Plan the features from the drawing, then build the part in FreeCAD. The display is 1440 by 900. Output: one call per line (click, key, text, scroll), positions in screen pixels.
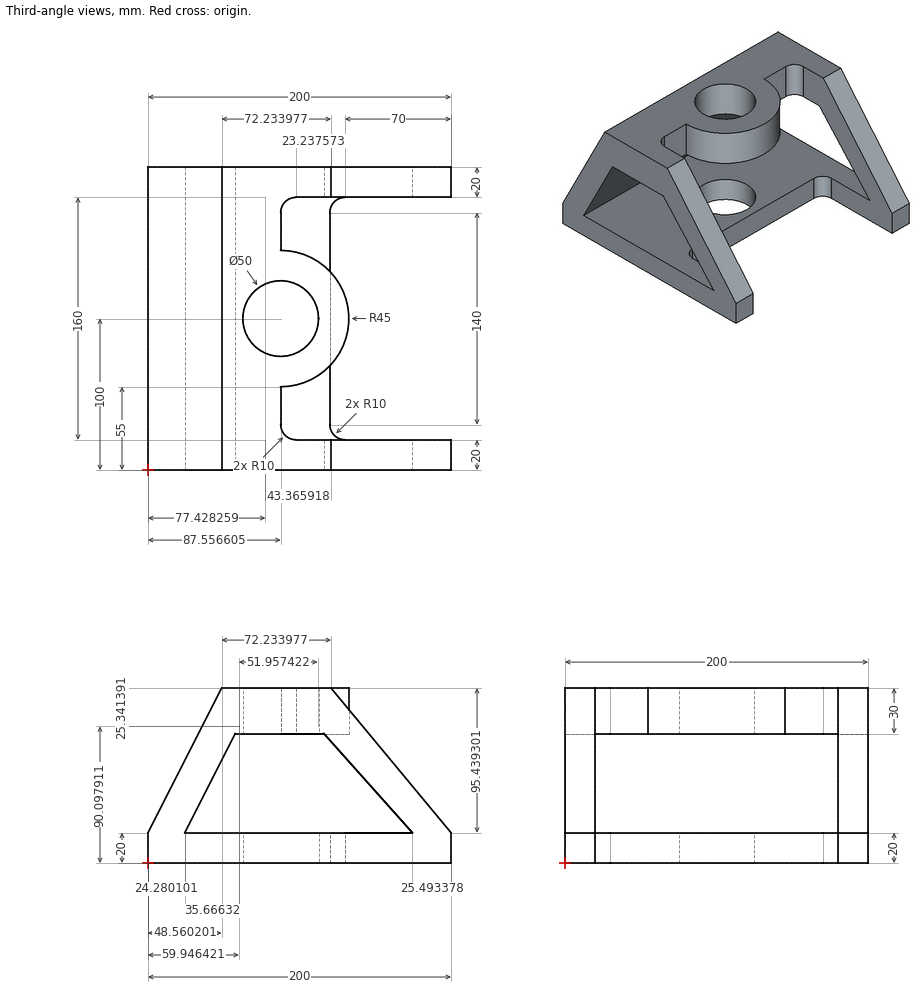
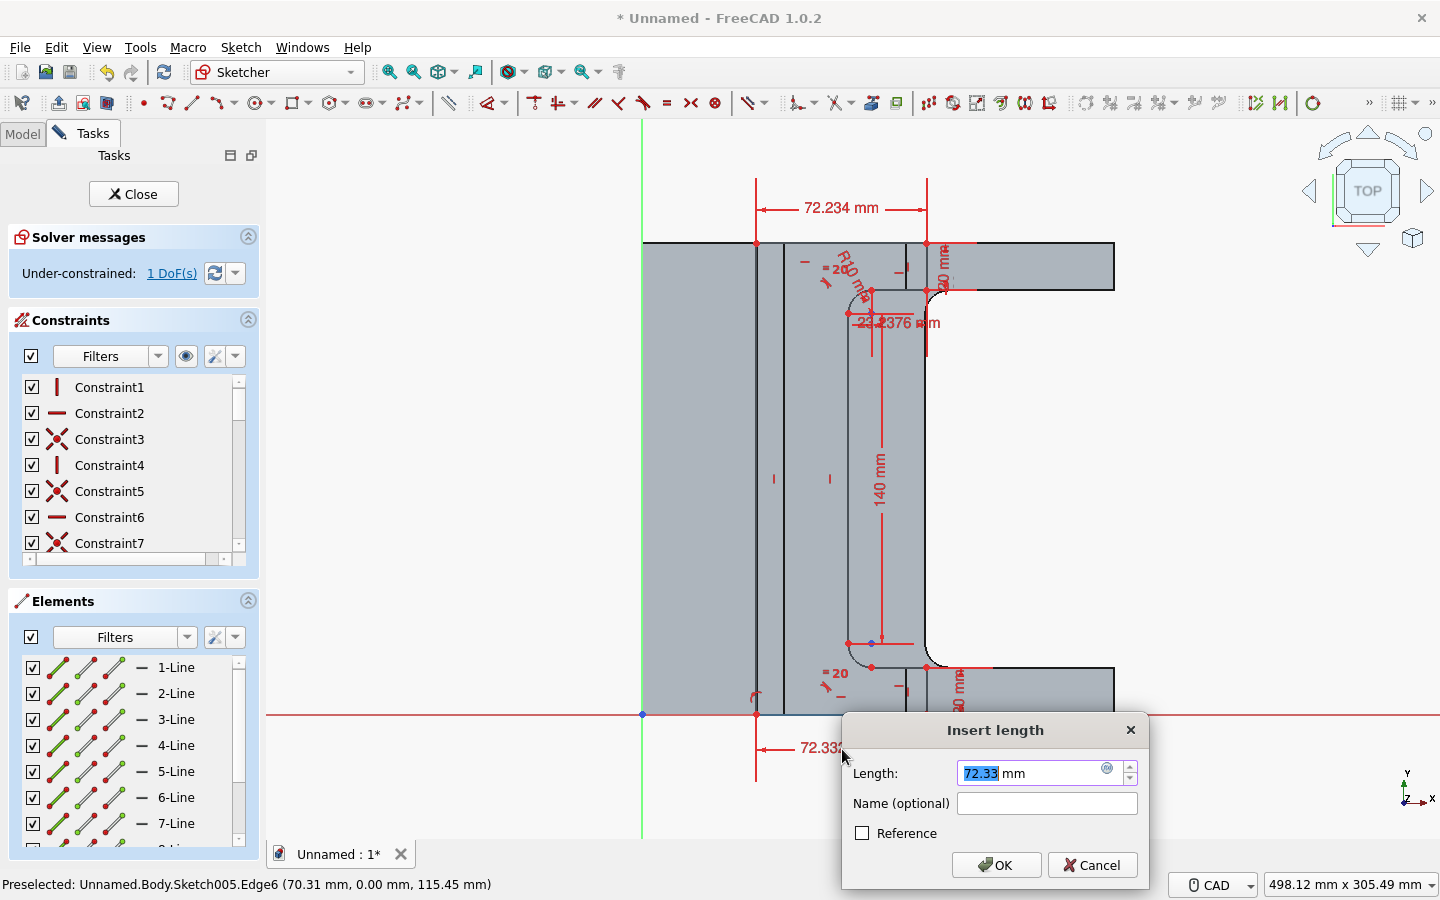
text(72.233977)
key(Return)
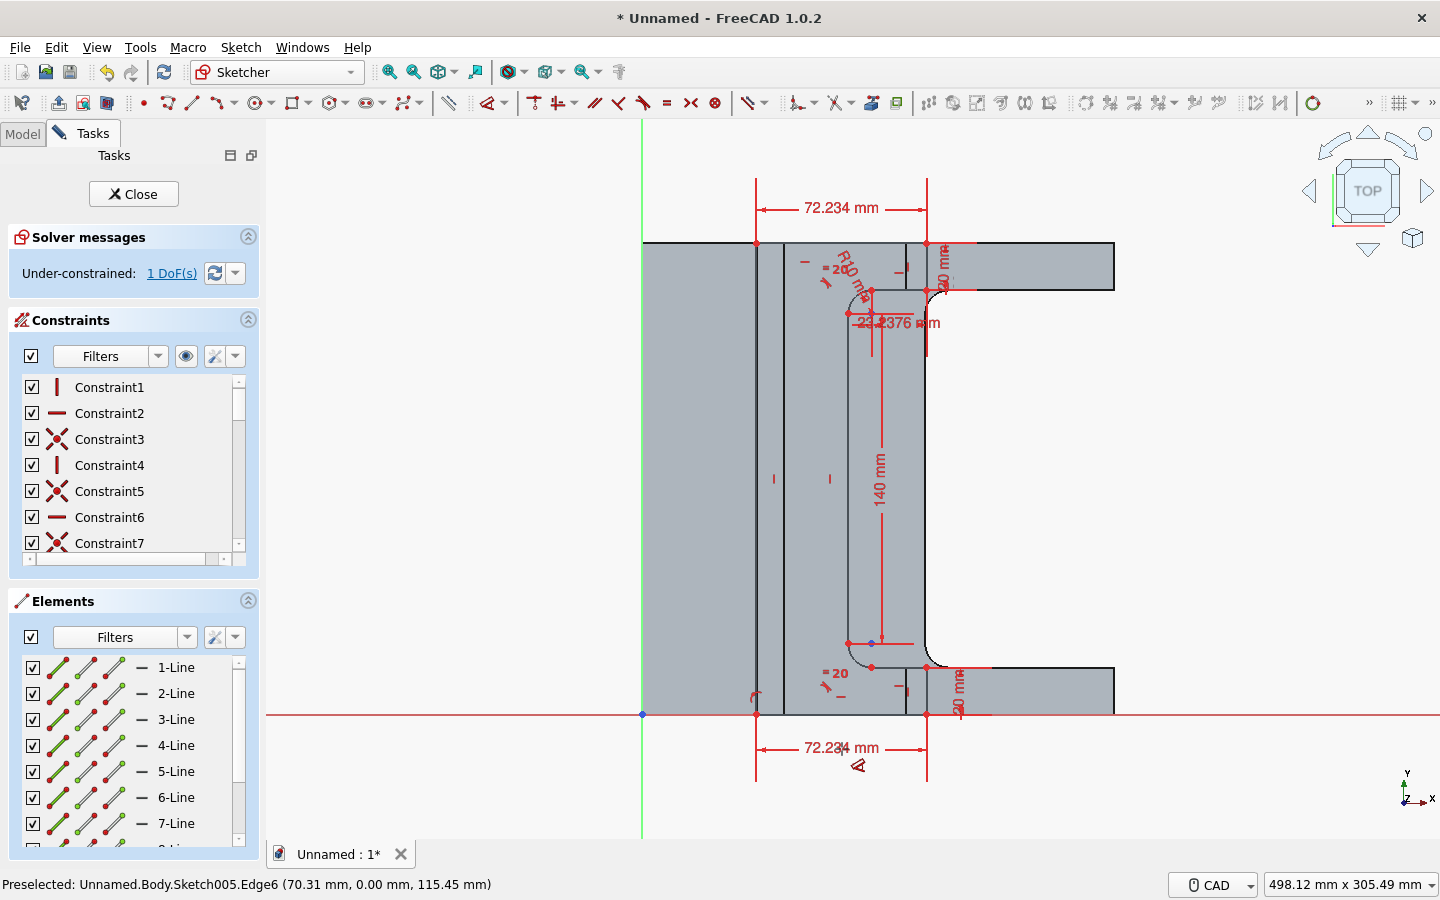
click(848, 644)
click(745, 749)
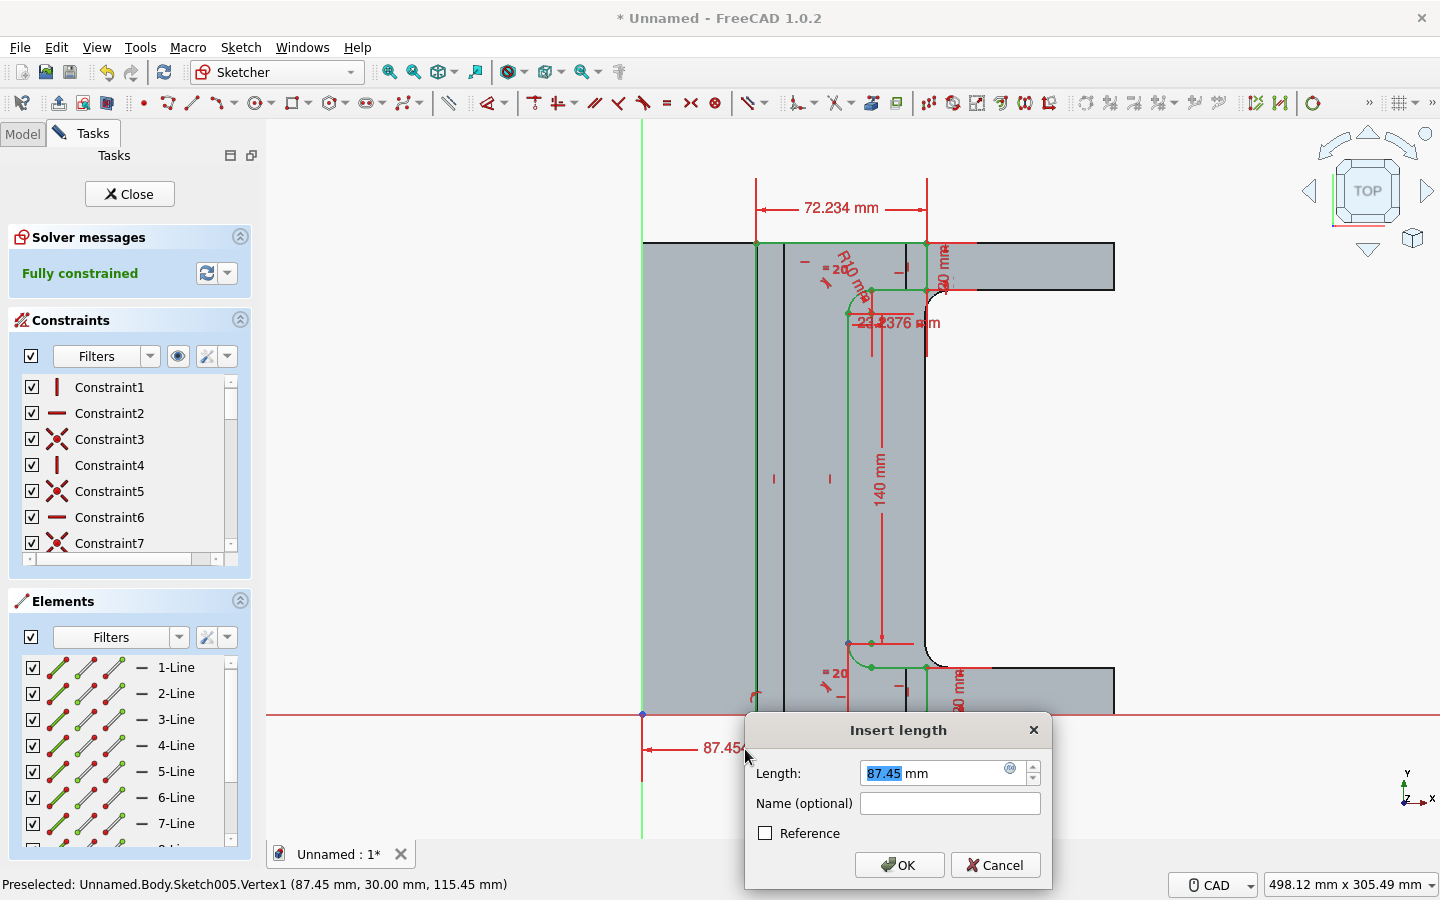
text(87.556605)
key(Return)
key(Escape)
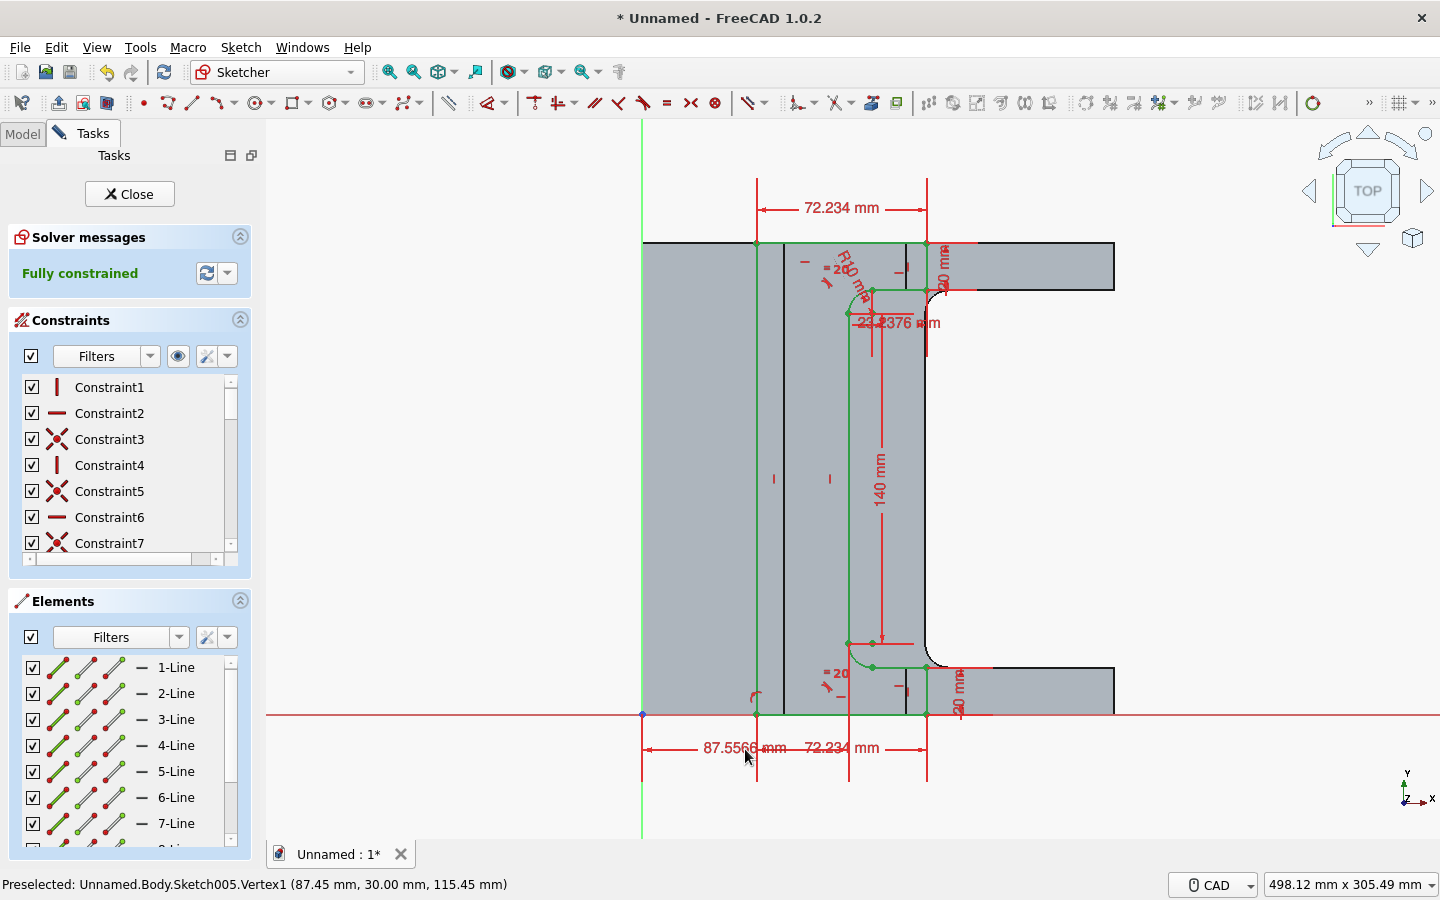
click(130, 194)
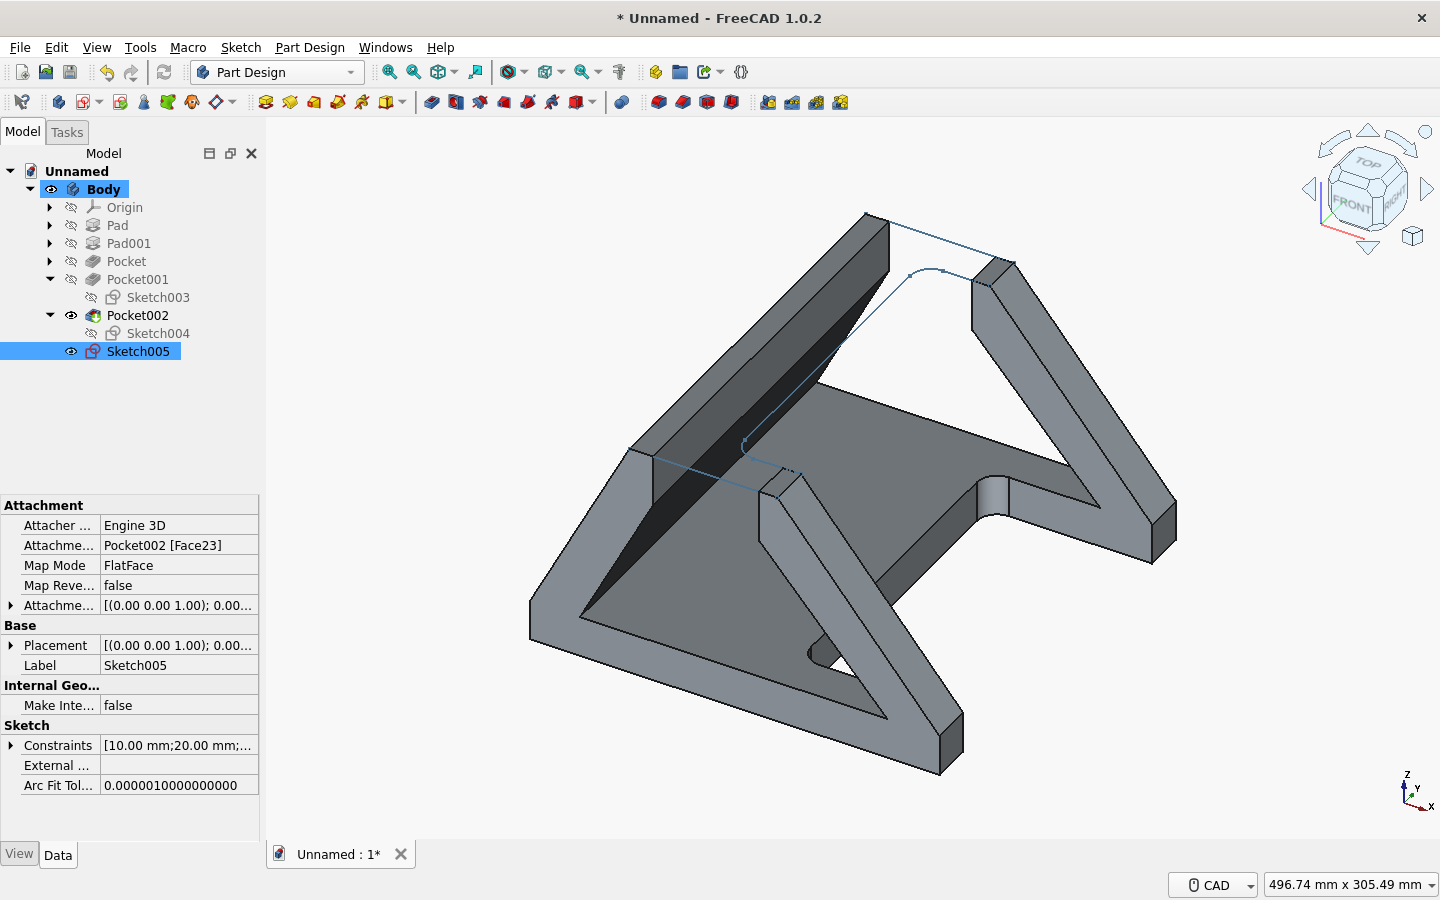
click(266, 102)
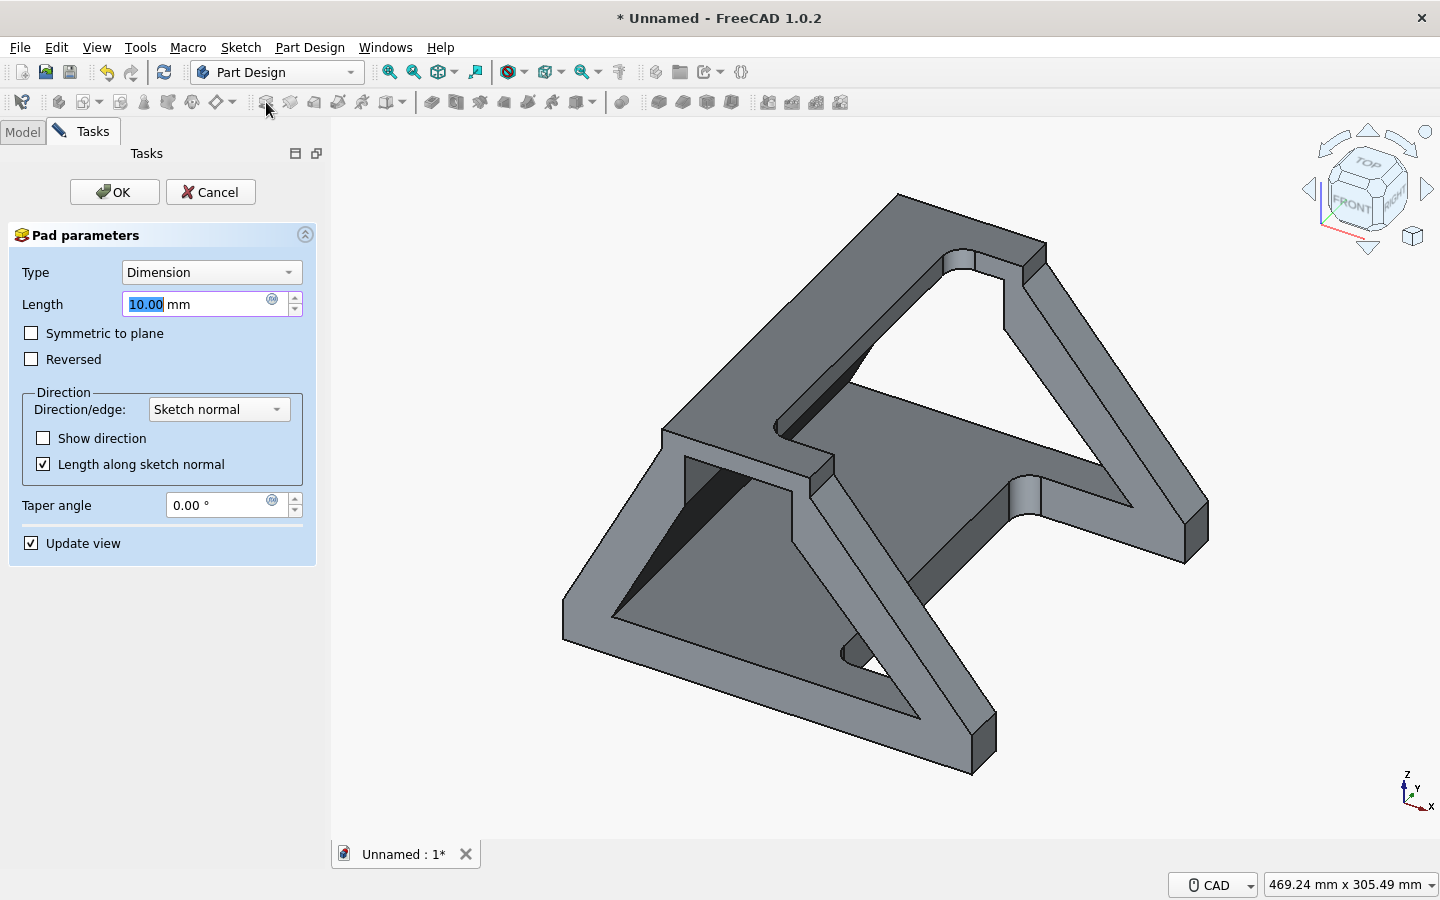
text(30)
key(Tab)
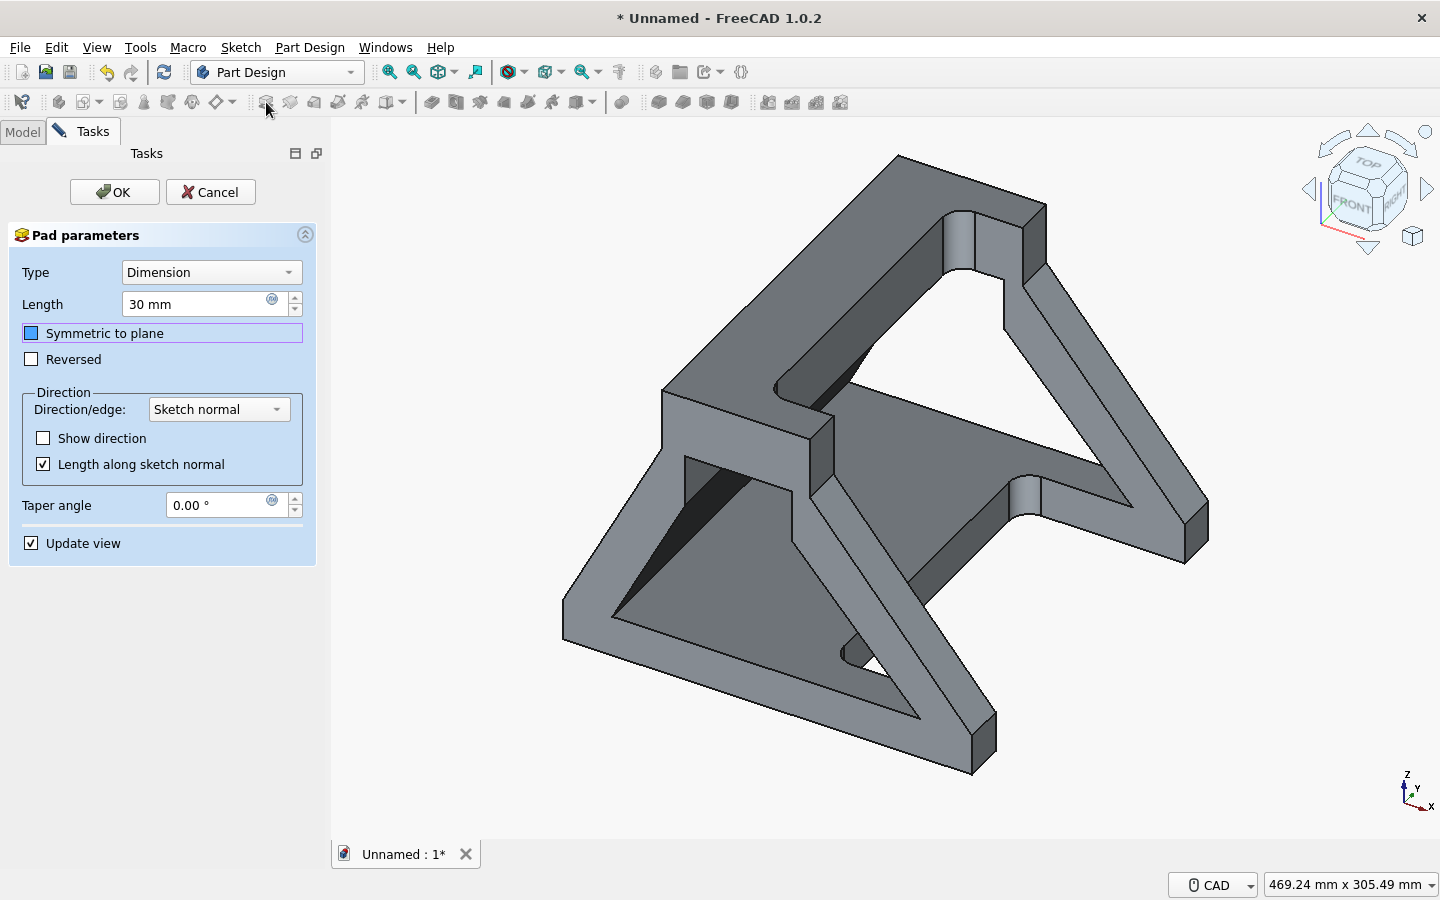
click(30, 359)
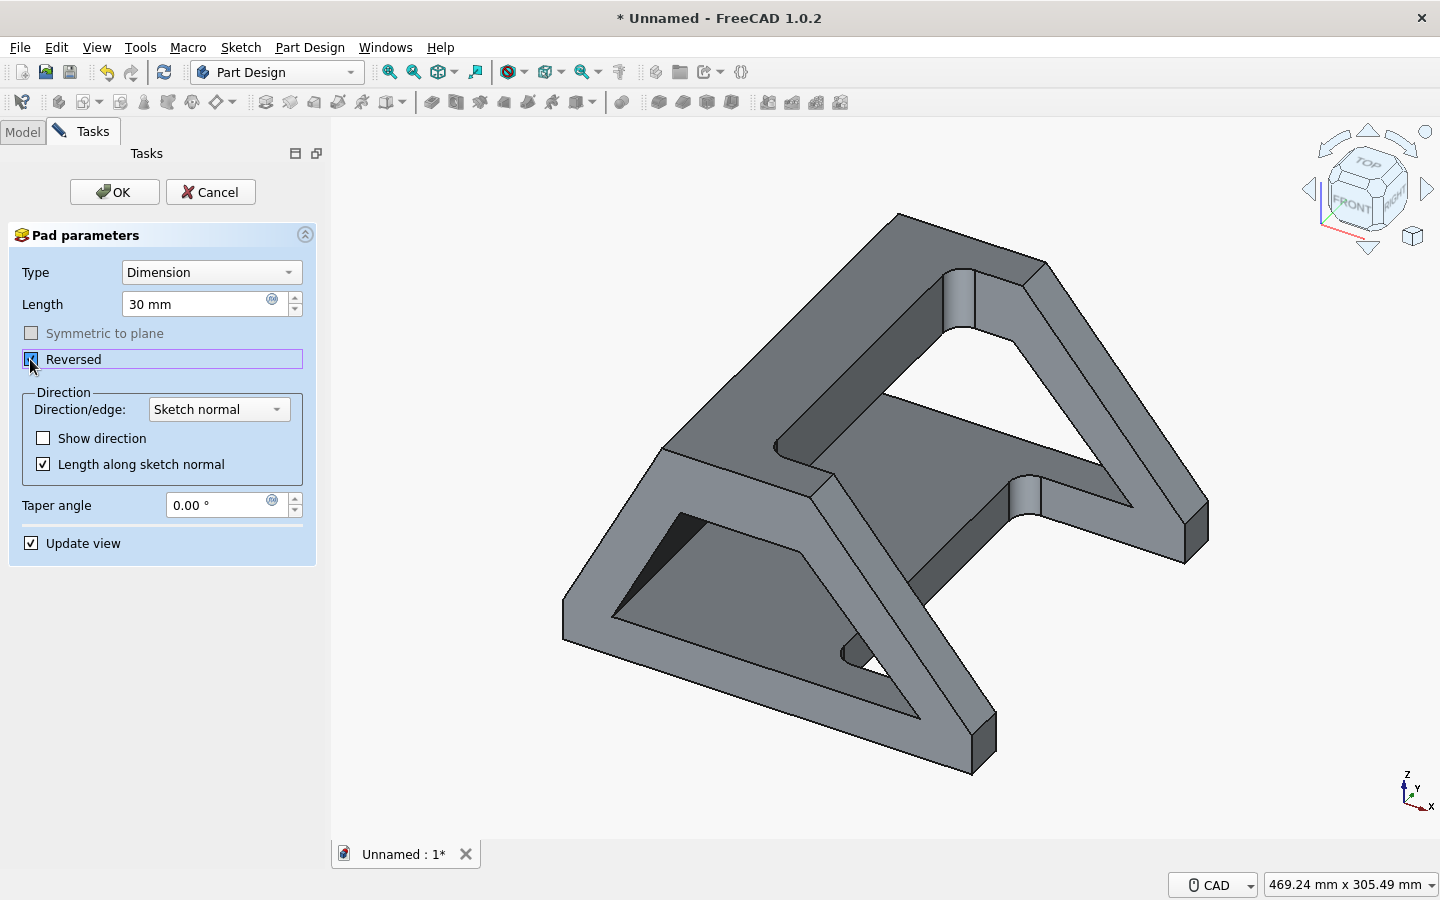
click(115, 192)